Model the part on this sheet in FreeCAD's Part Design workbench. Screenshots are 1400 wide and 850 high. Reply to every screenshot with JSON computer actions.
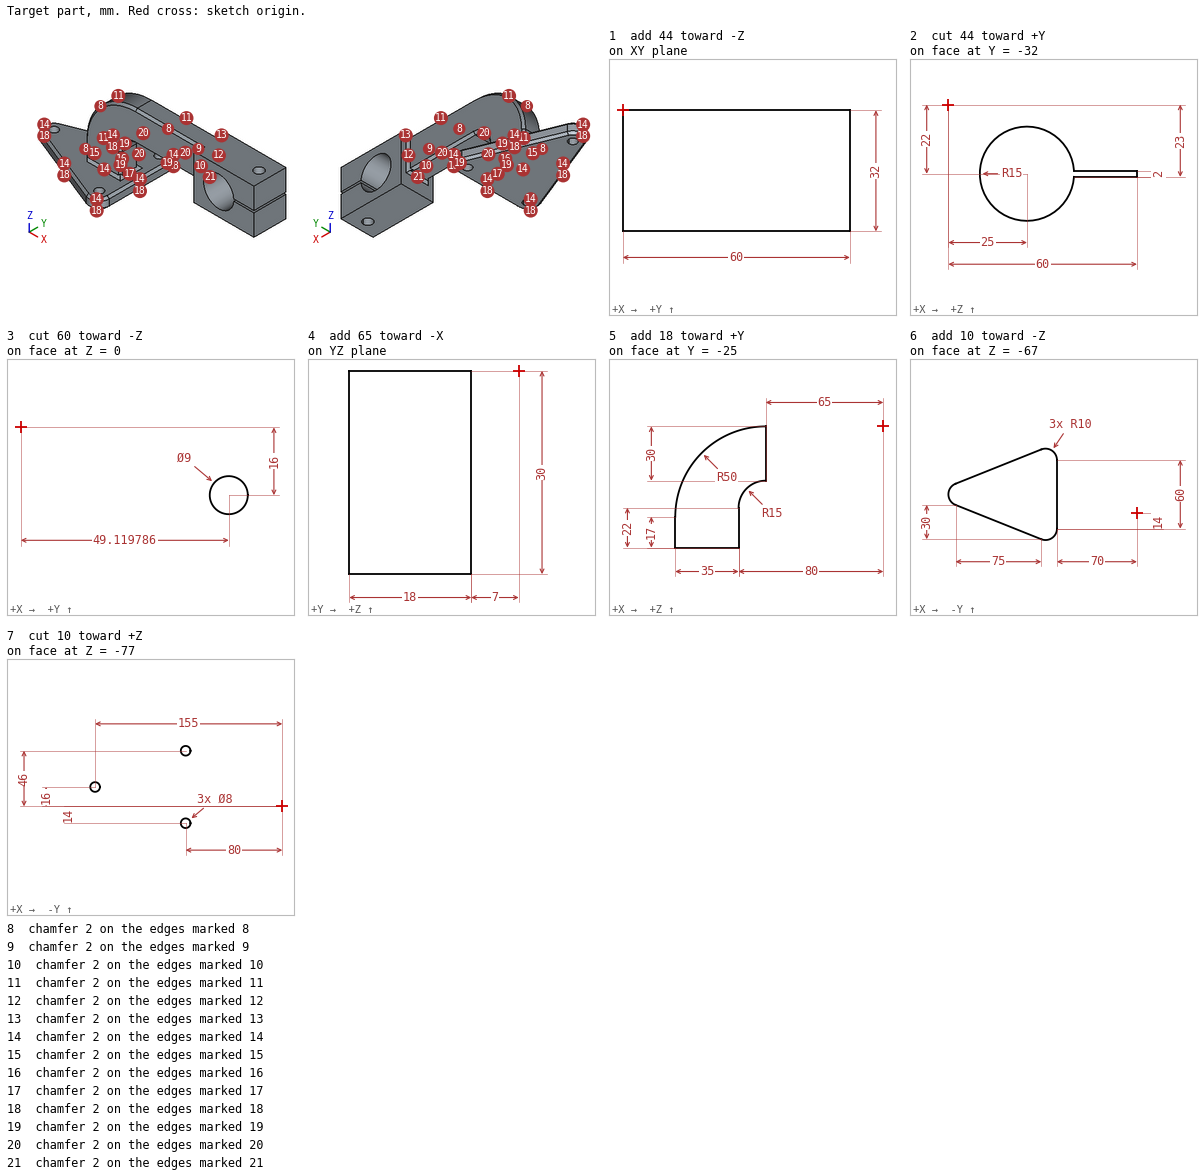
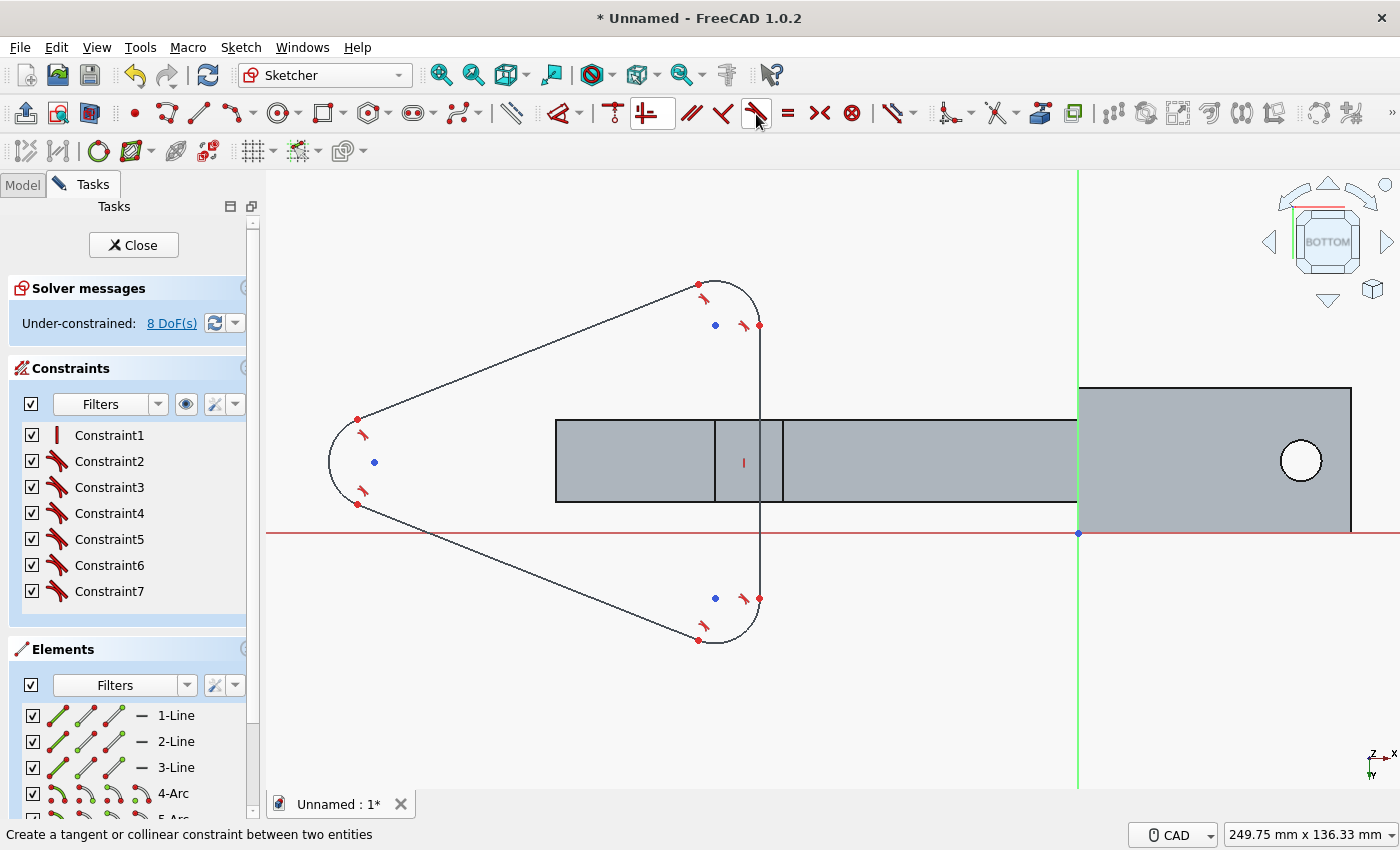
{"action": "left_click", "coordinate": [724, 642]}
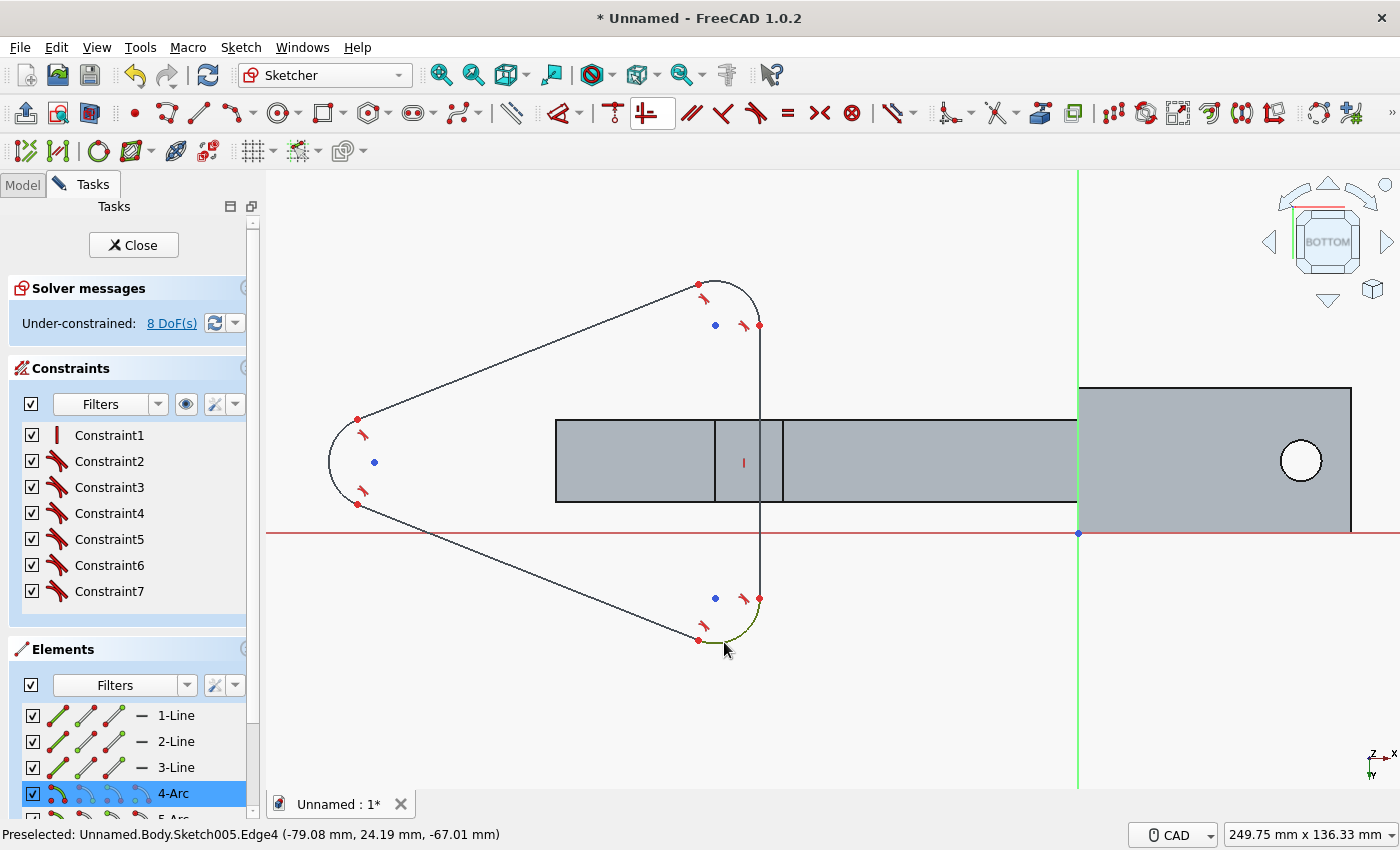
{"action": "left_click", "coordinate": [752, 301]}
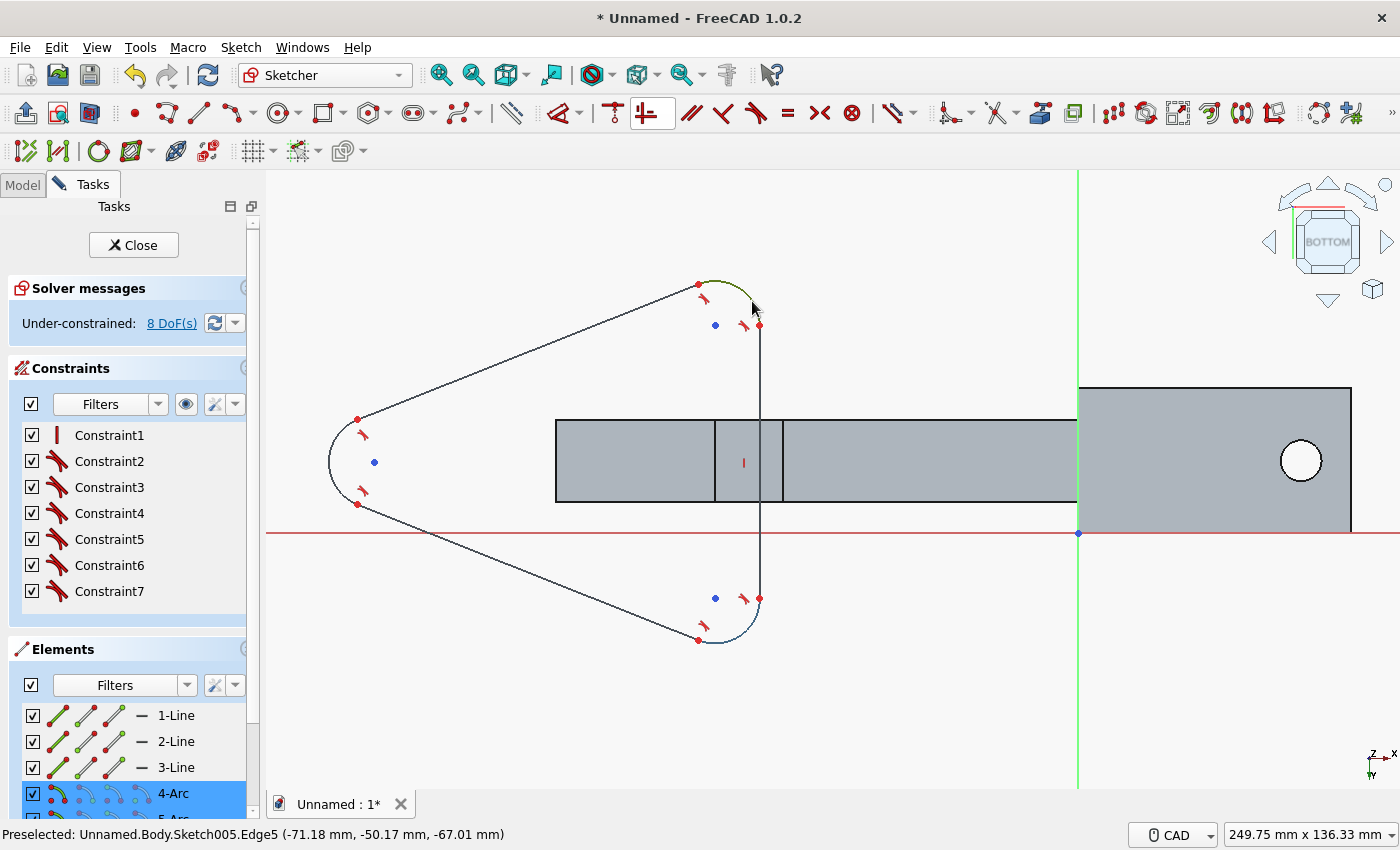
{"action": "left_click", "coordinate": [334, 441]}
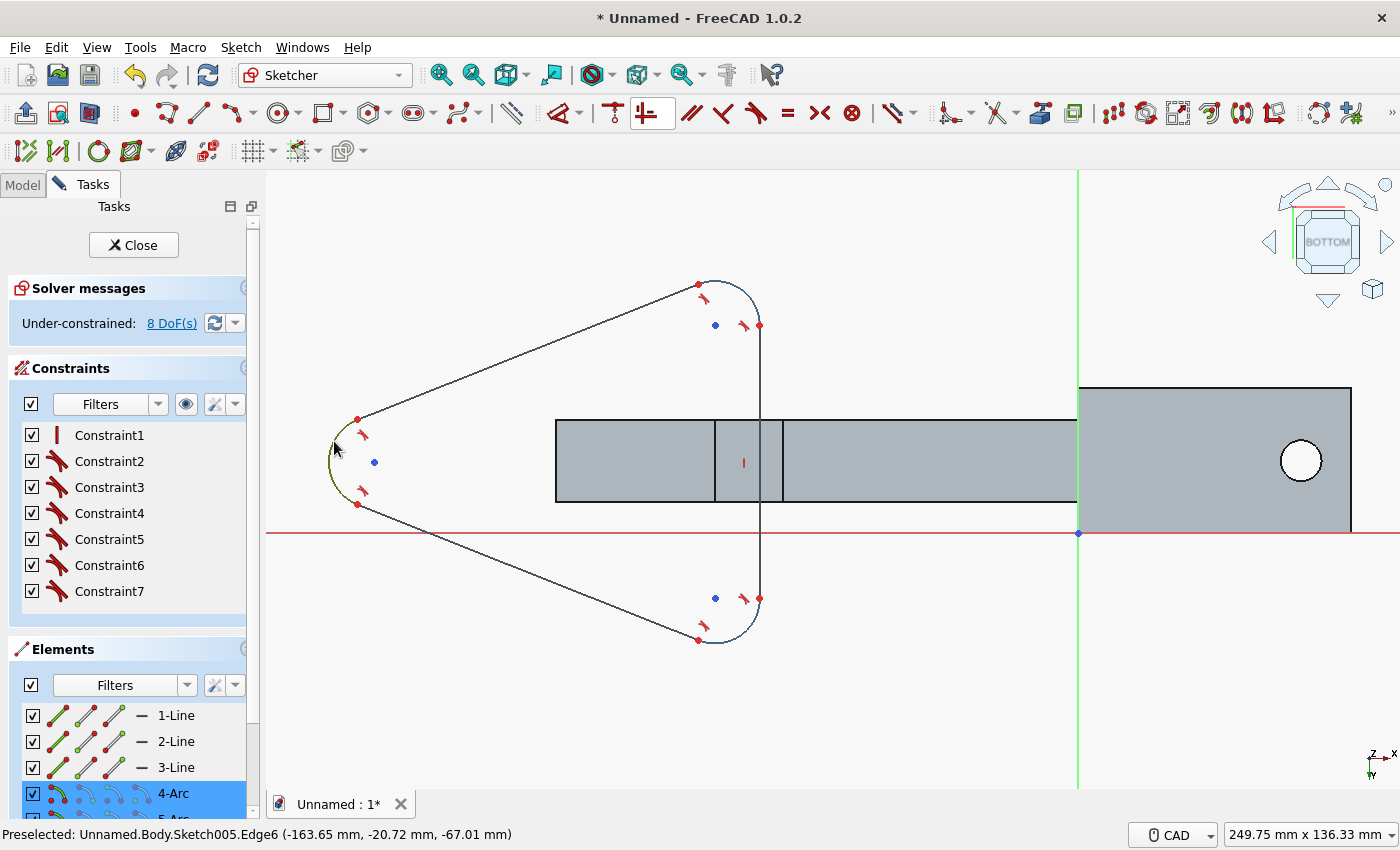
{"action": "left_click", "coordinate": [788, 114]}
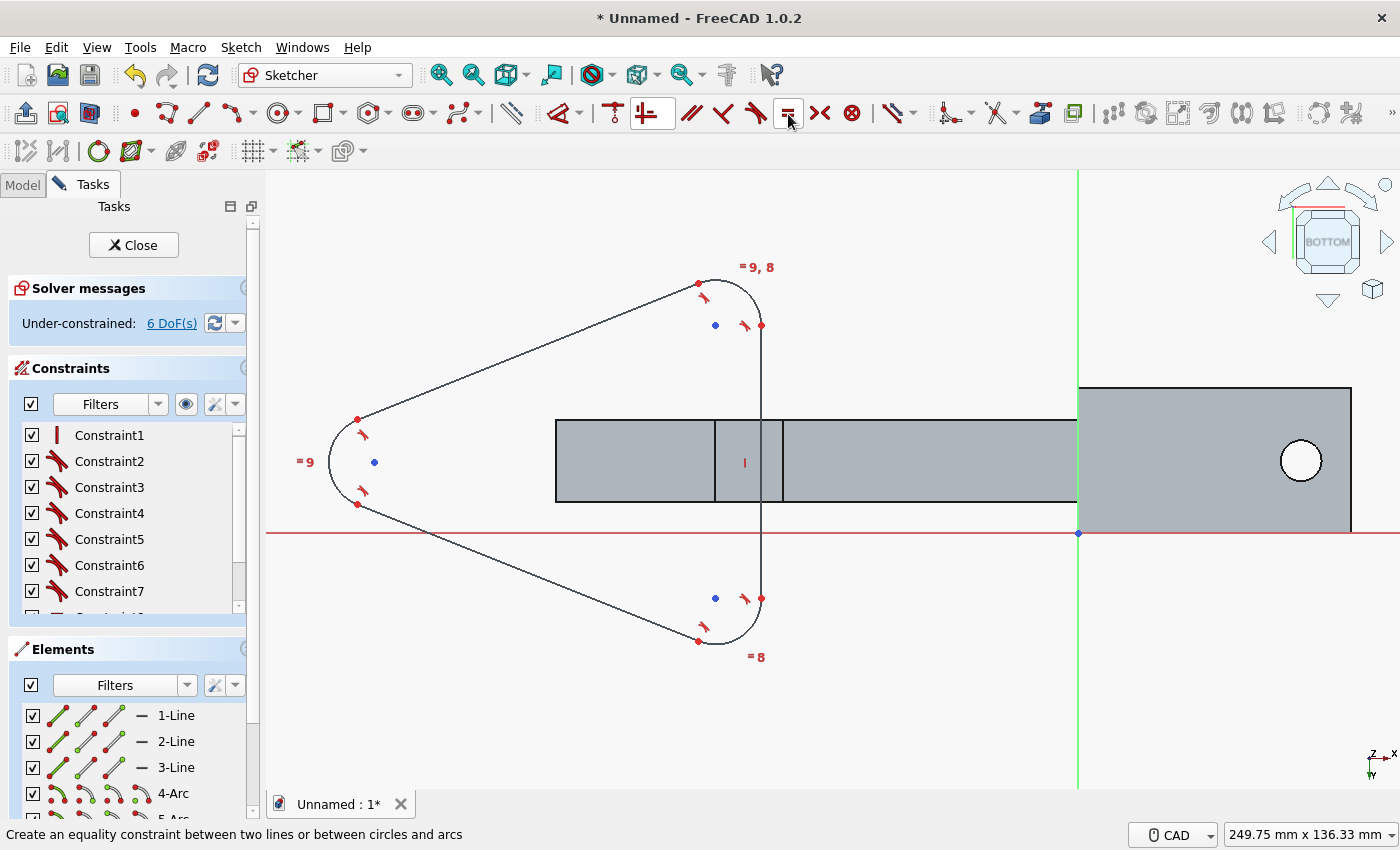
{"action": "left_click", "coordinate": [558, 114]}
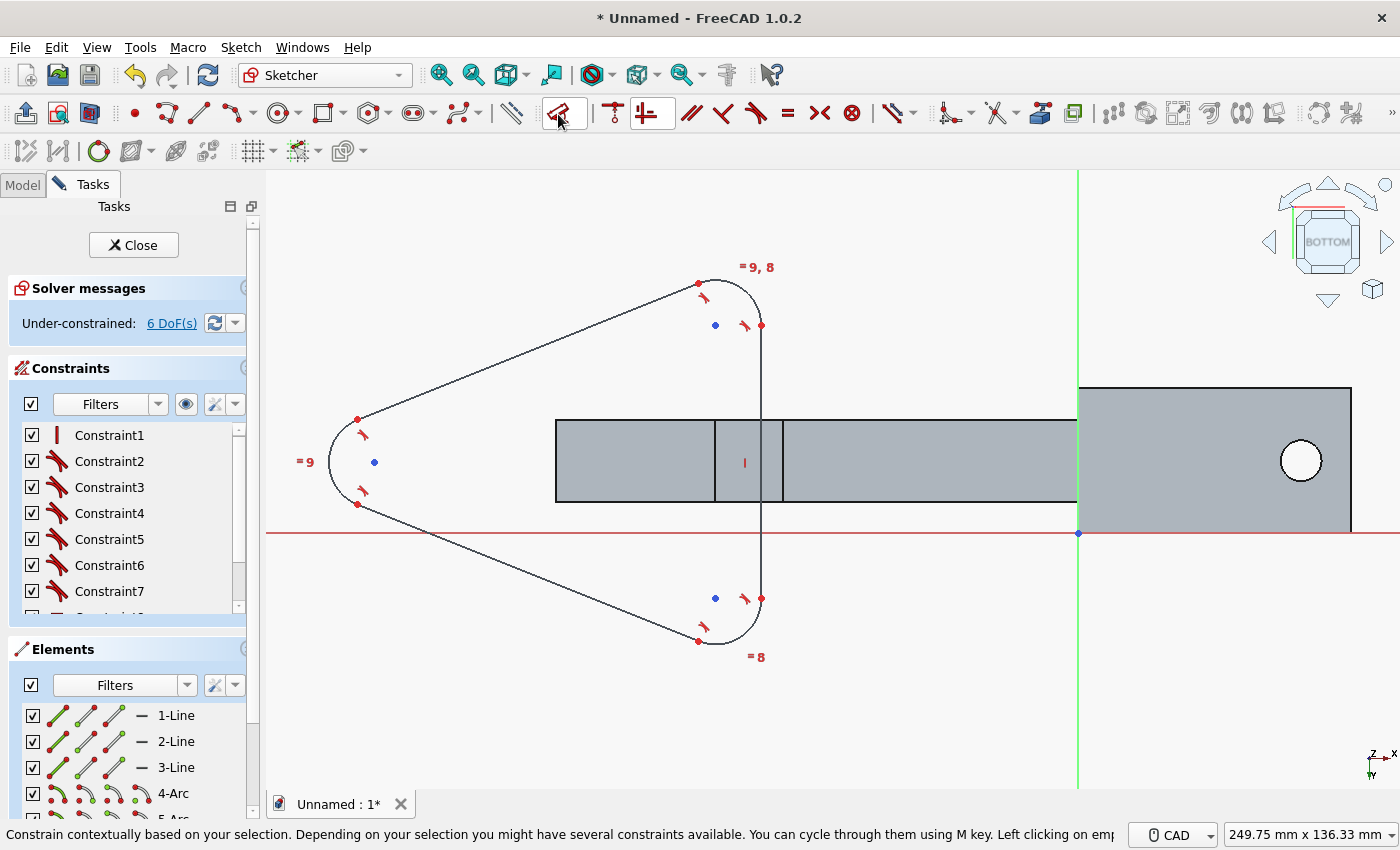
{"action": "left_click", "coordinate": [725, 643]}
{"action": "left_click", "coordinate": [732, 674]}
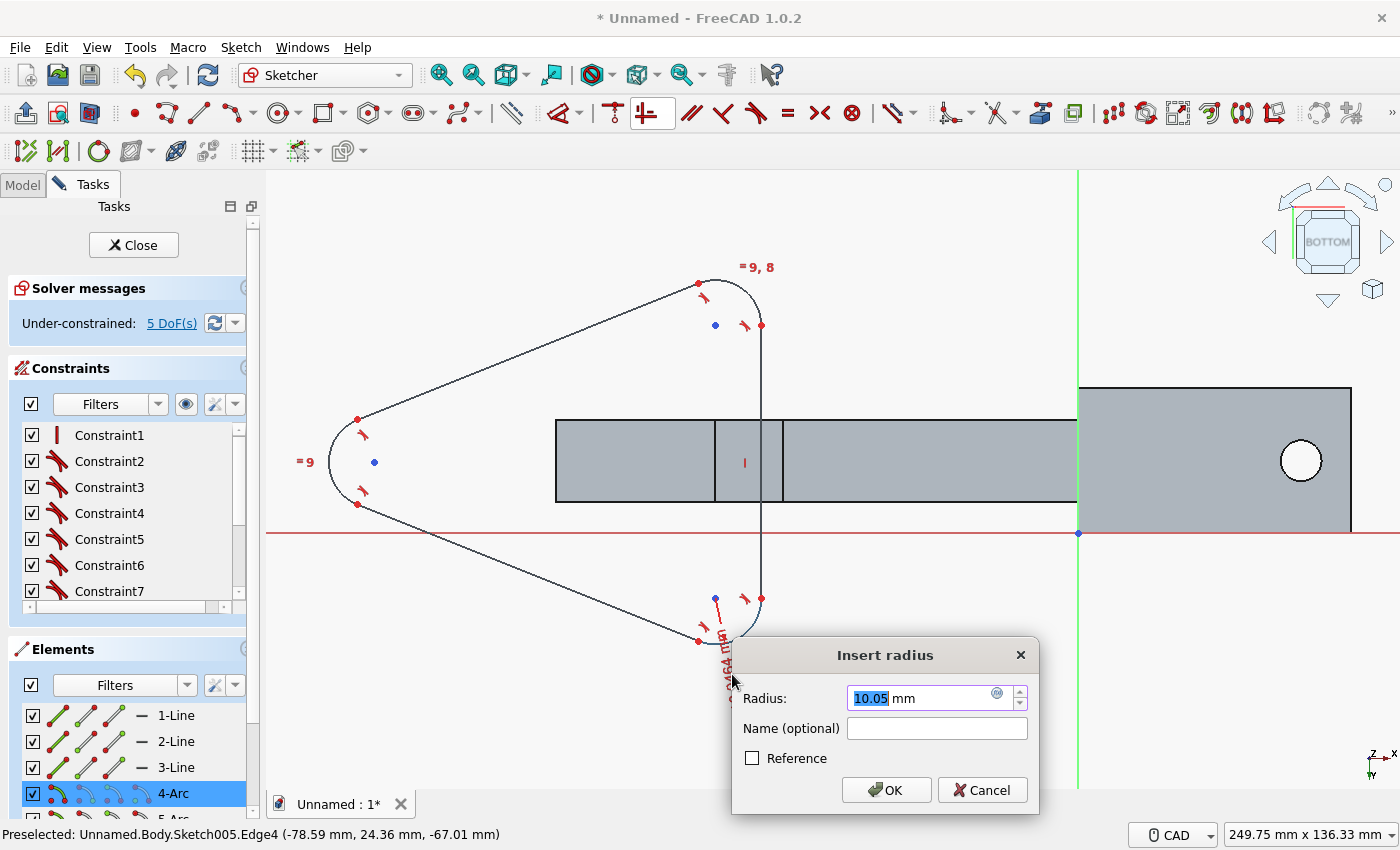
{"action": "type", "text": "10"}
{"action": "key", "text": "Return"}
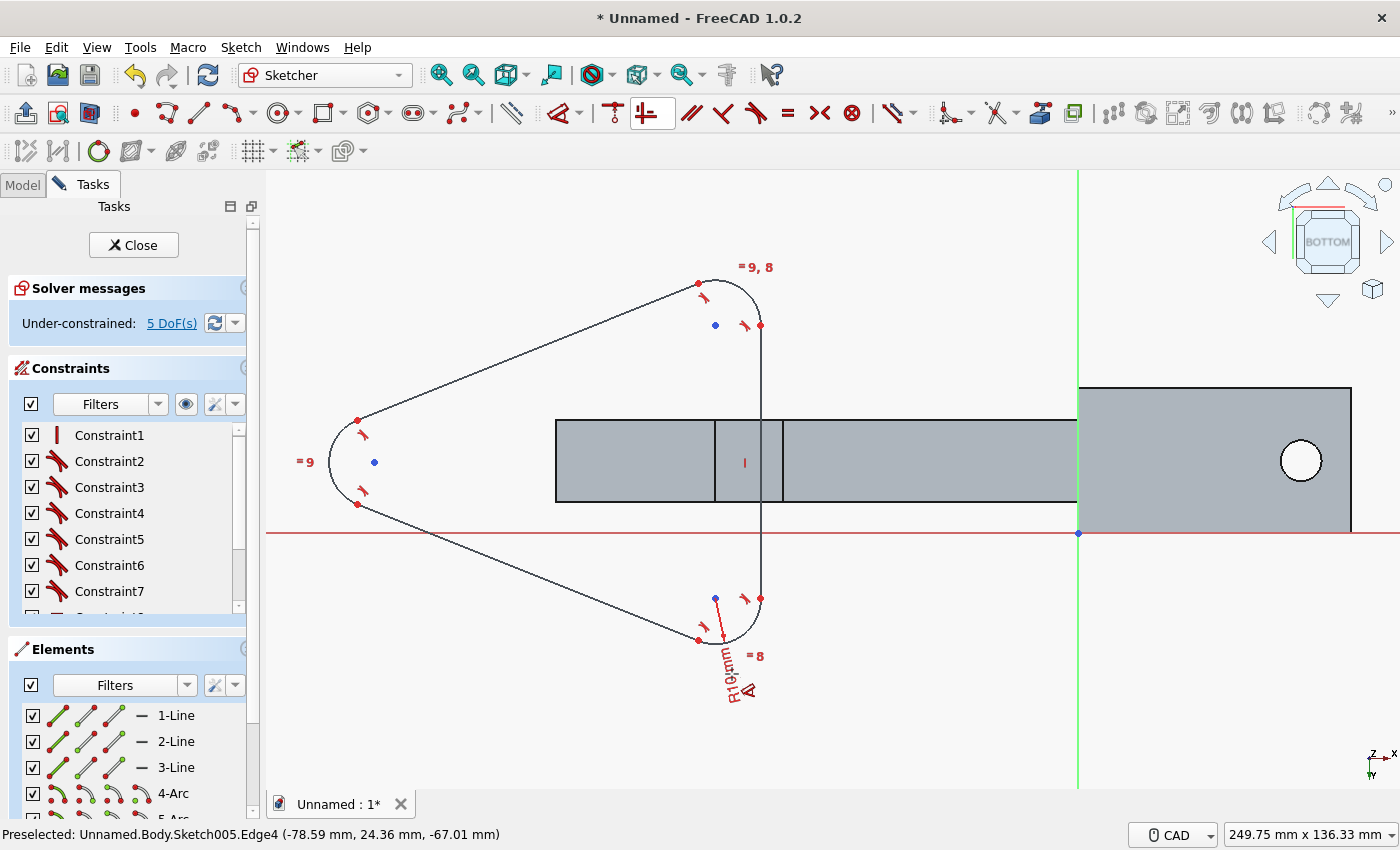
{"action": "left_click", "coordinate": [761, 517]}
{"action": "left_click", "coordinate": [795, 462]}